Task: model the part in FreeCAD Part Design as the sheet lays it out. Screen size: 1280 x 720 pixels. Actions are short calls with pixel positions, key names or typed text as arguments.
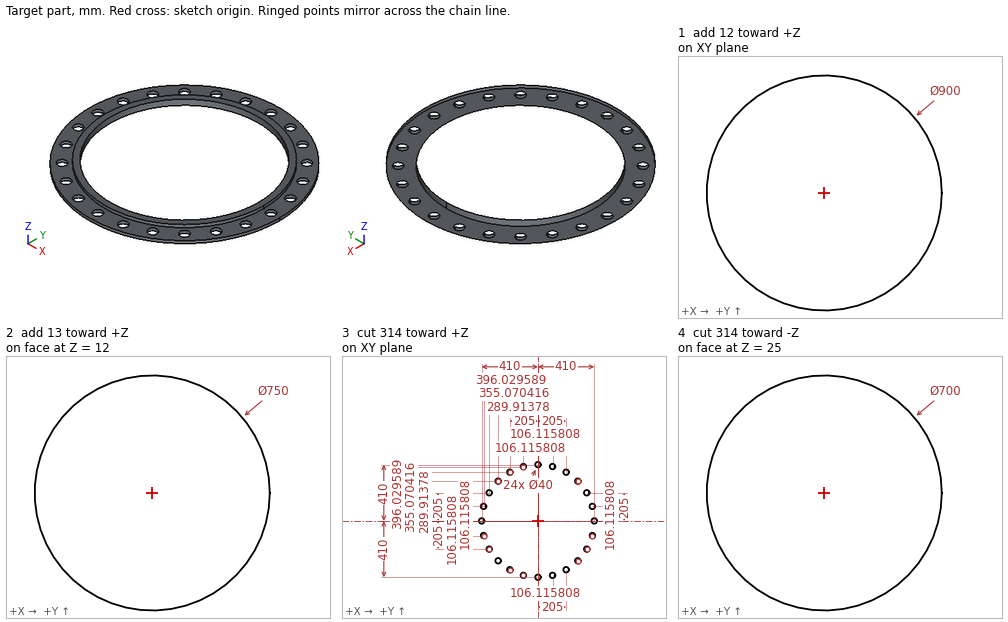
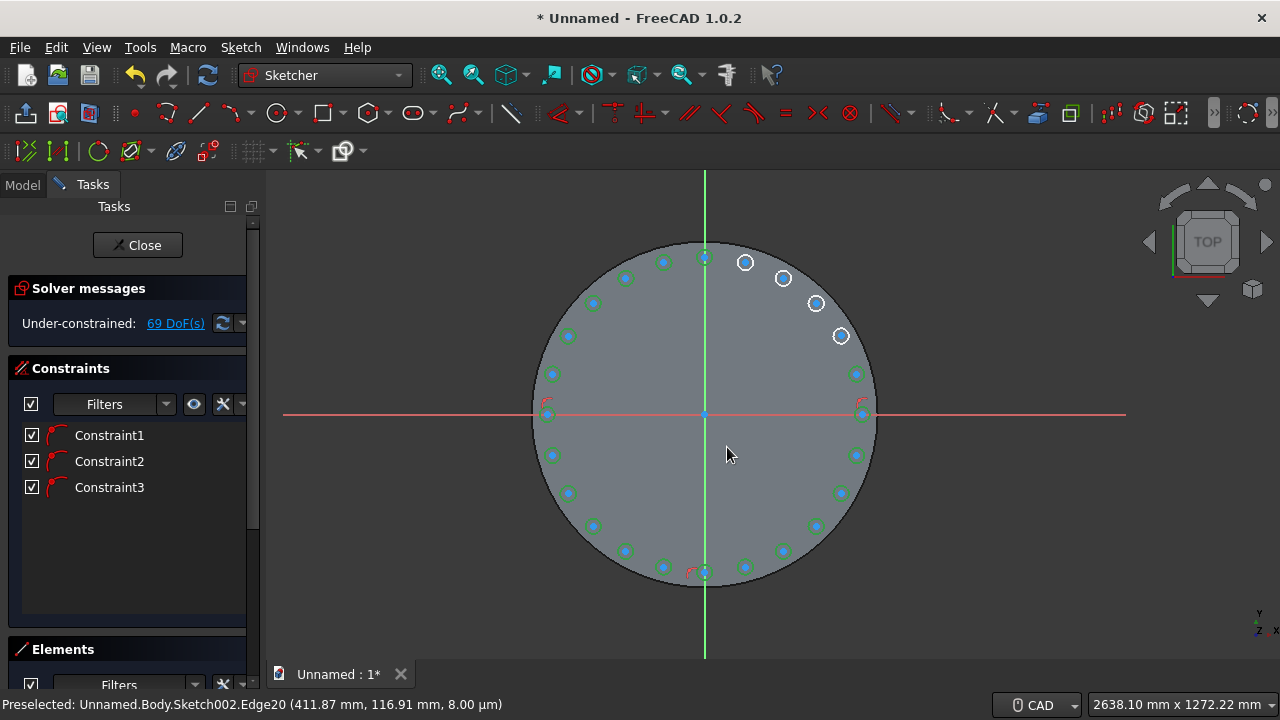
scroll(847, 331, up, 3)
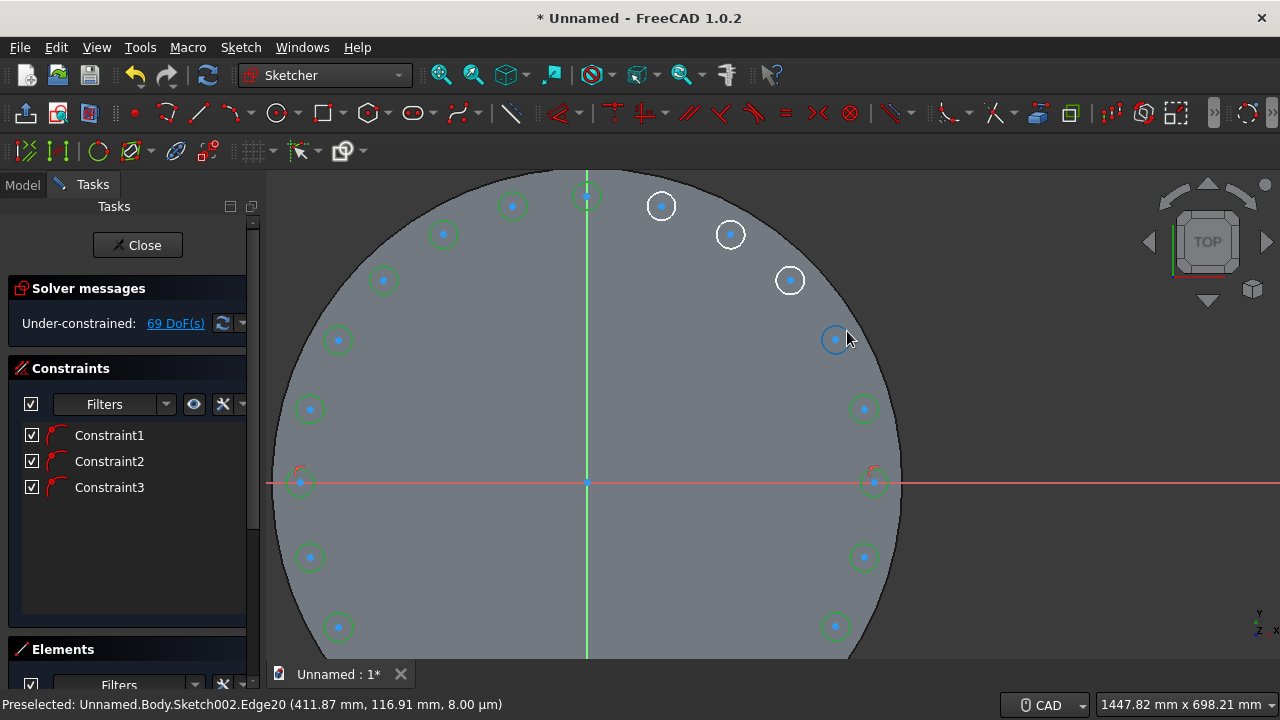
click(846, 330)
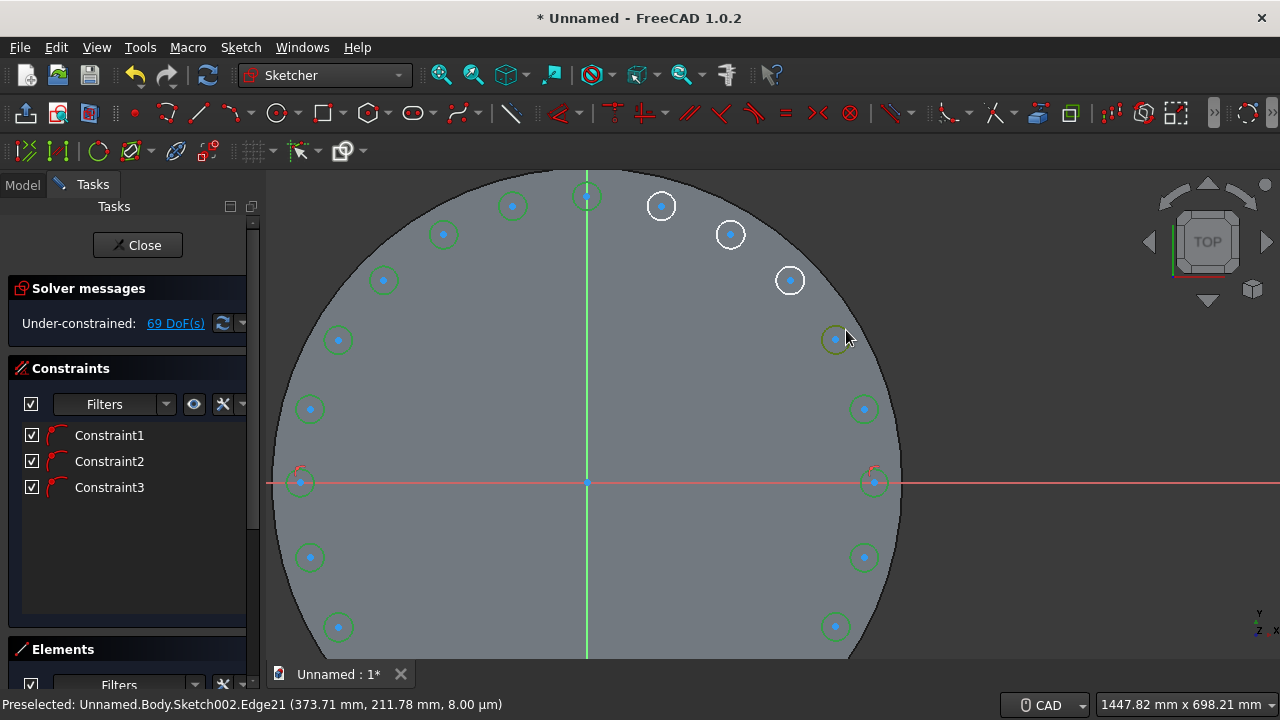
click(800, 271)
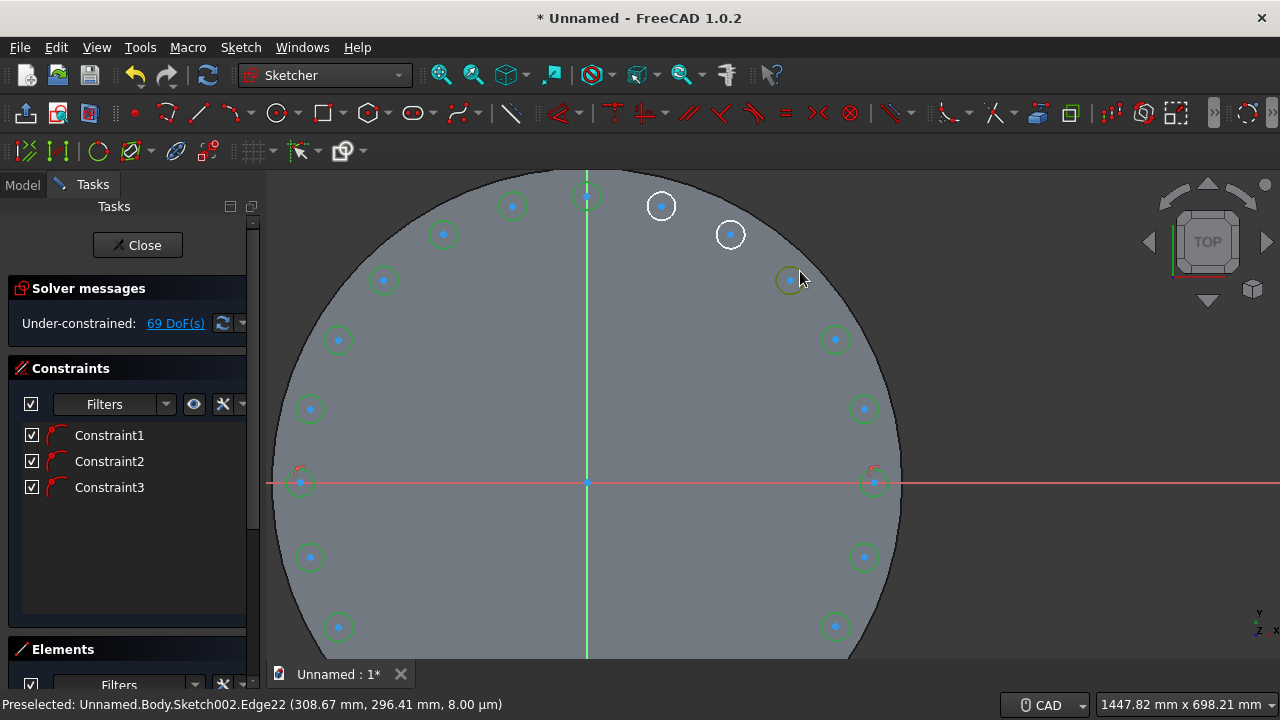
click(741, 225)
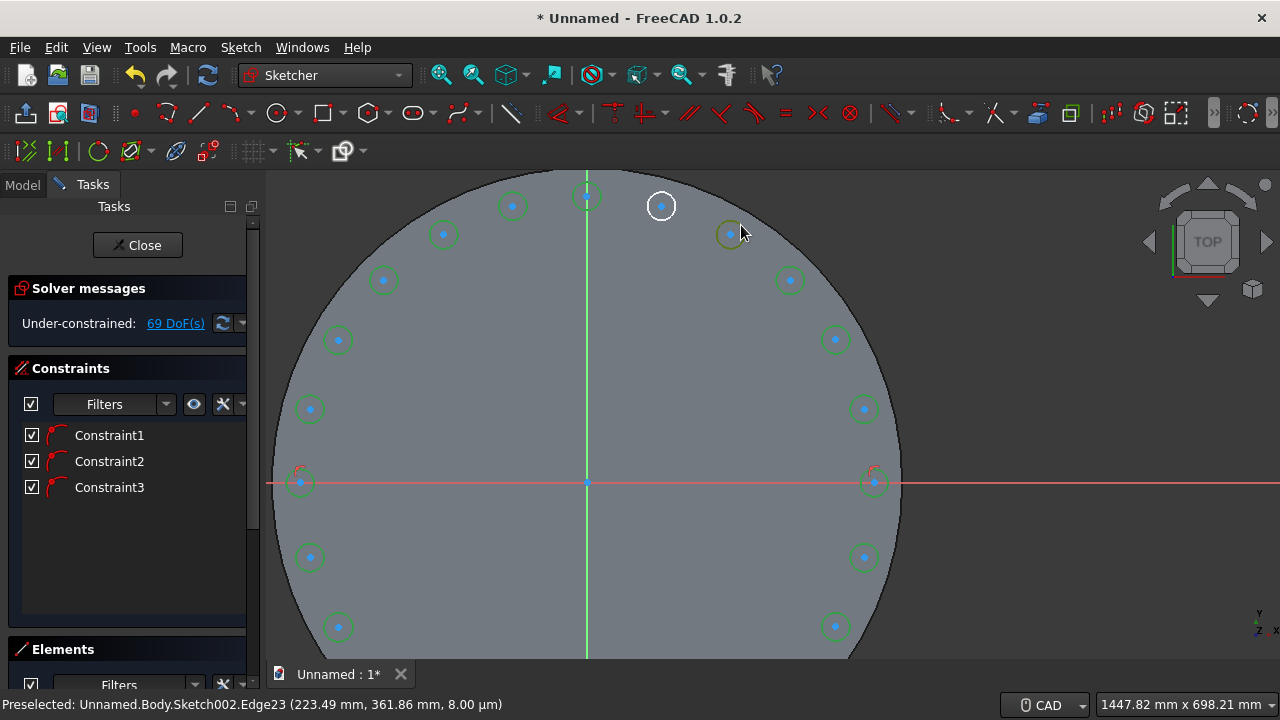
click(652, 216)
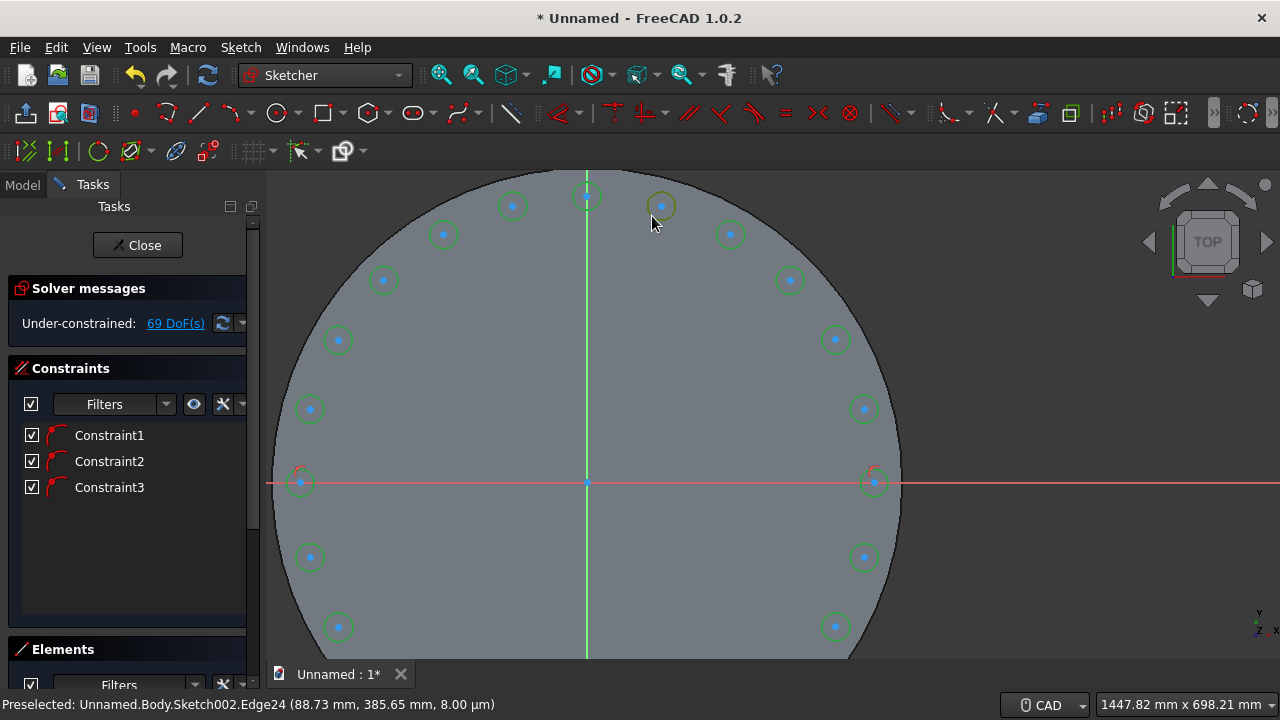
click(786, 114)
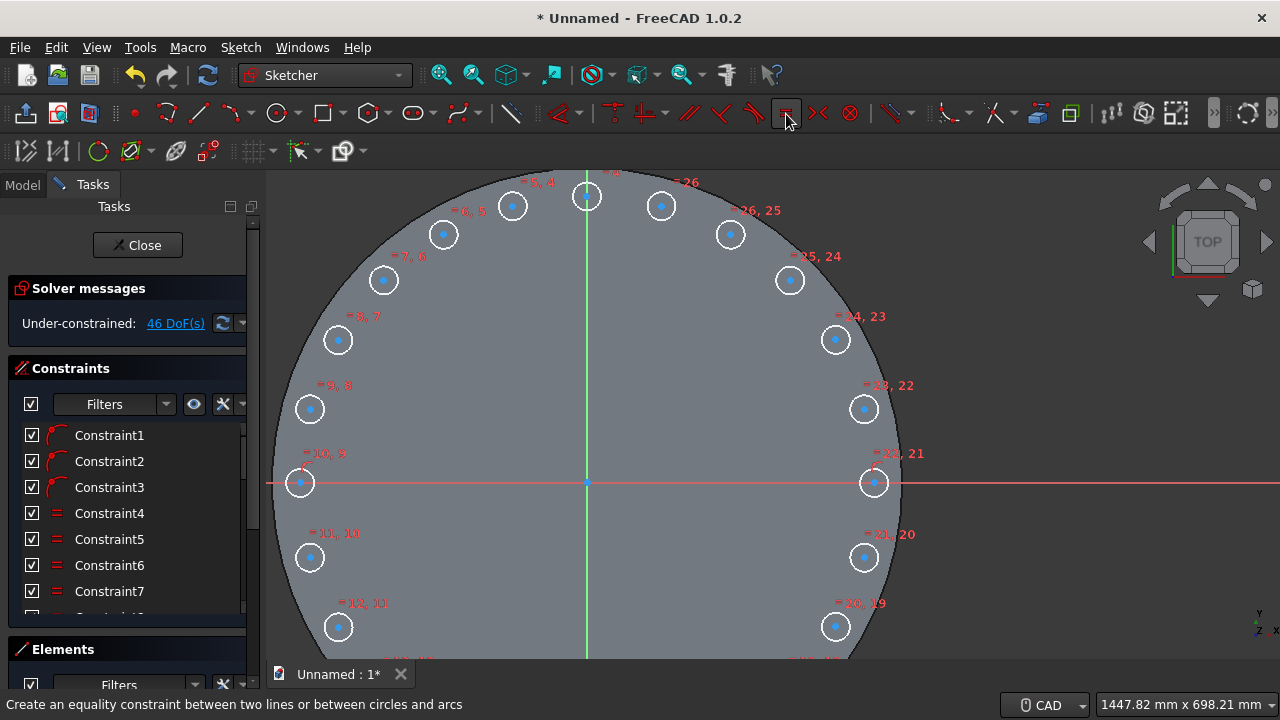
scroll(847, 331, down, 3)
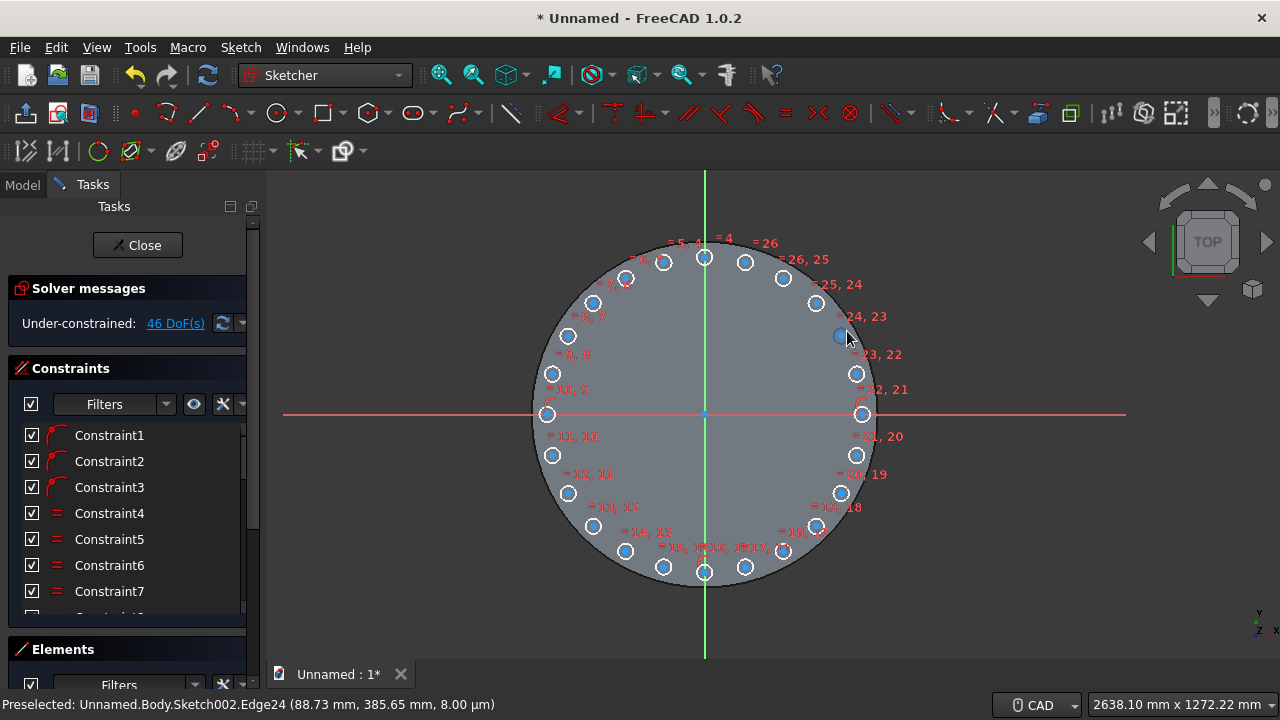
click(705, 257)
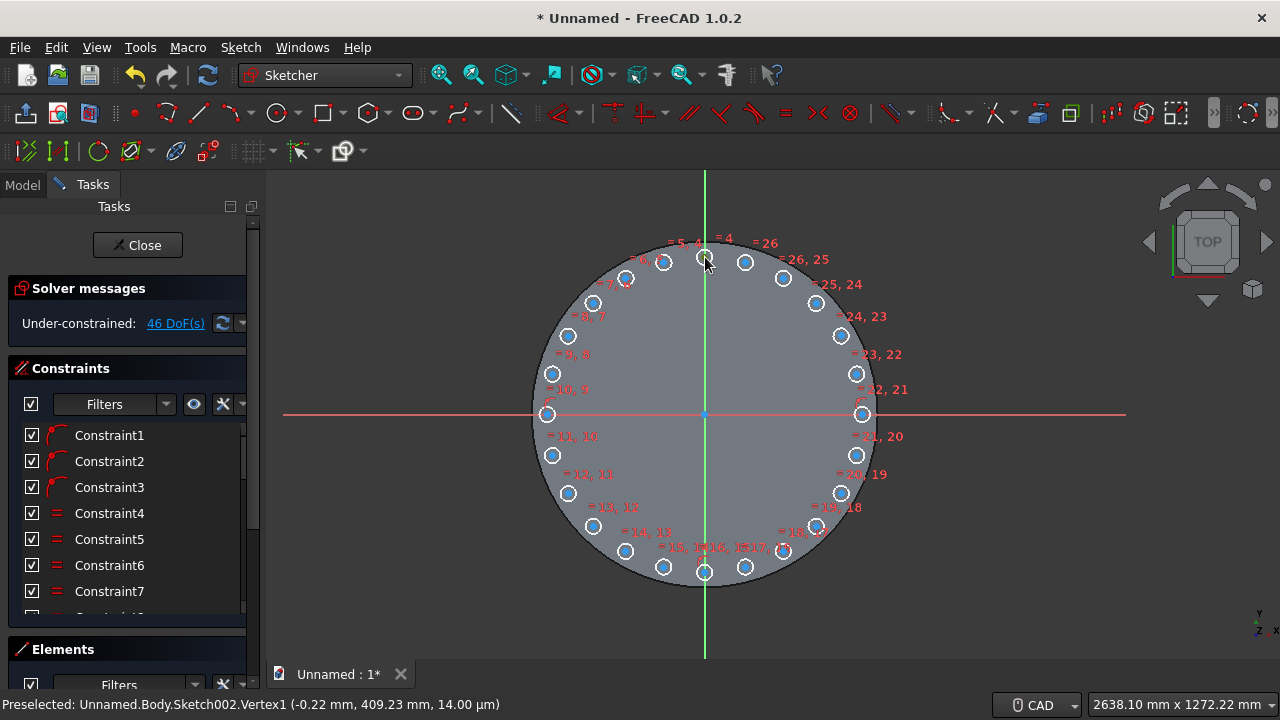
click(705, 507)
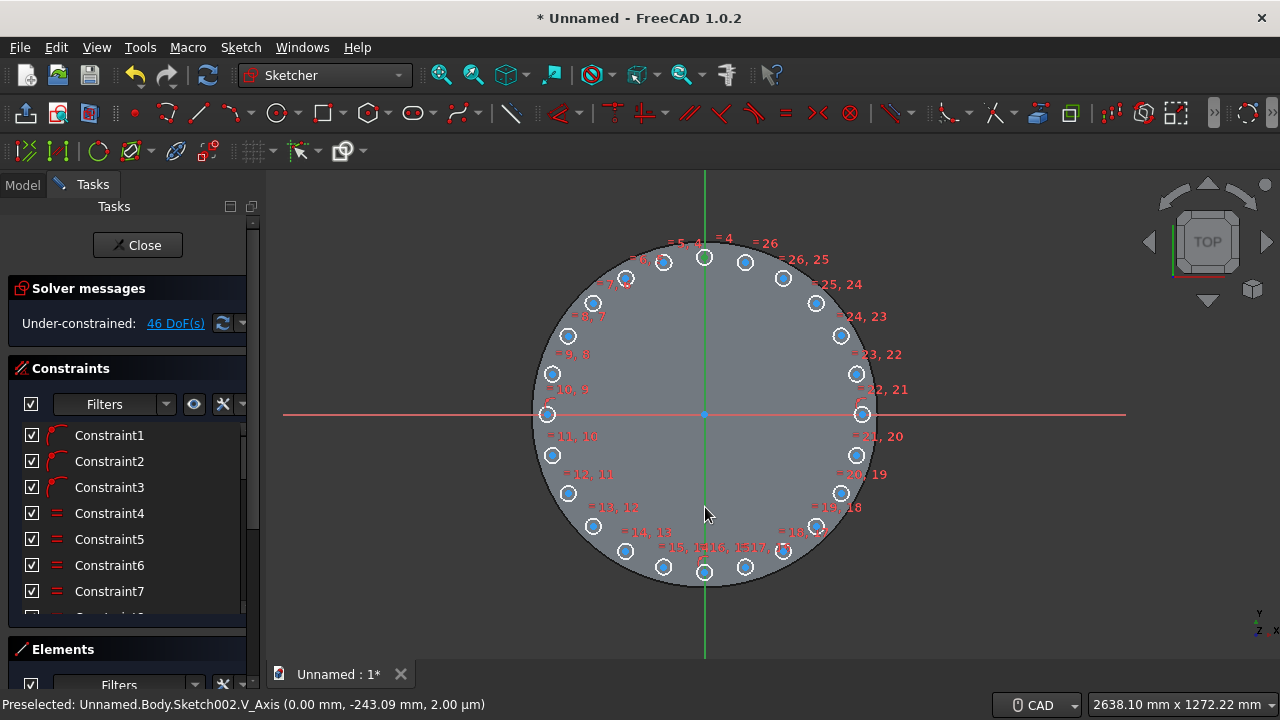
click(614, 114)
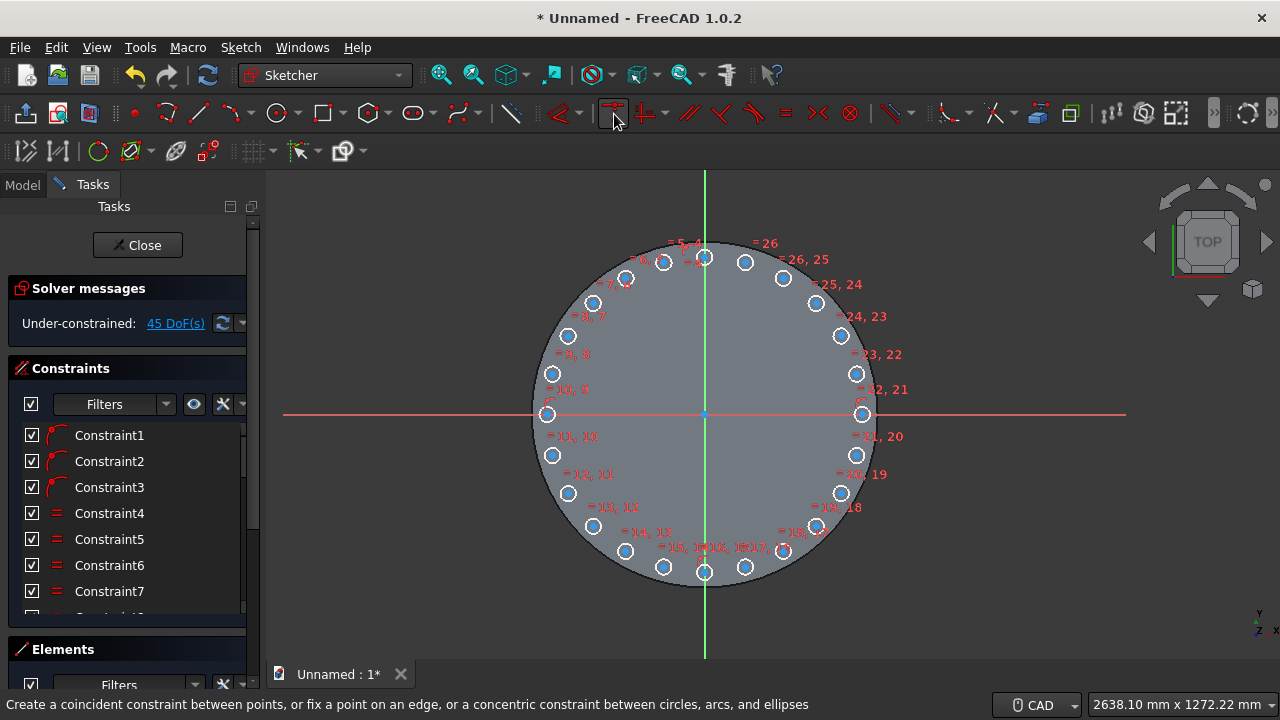
click(553, 374)